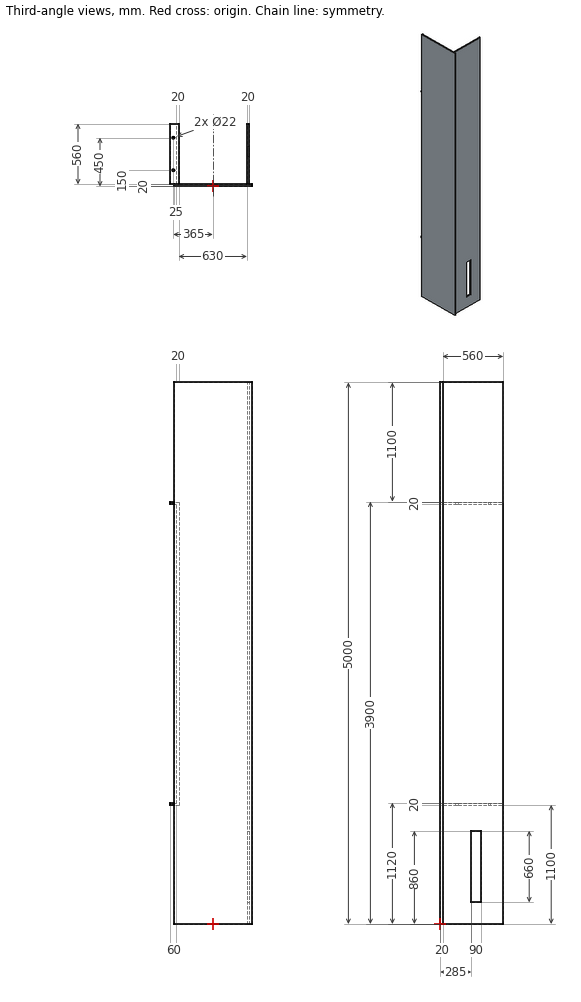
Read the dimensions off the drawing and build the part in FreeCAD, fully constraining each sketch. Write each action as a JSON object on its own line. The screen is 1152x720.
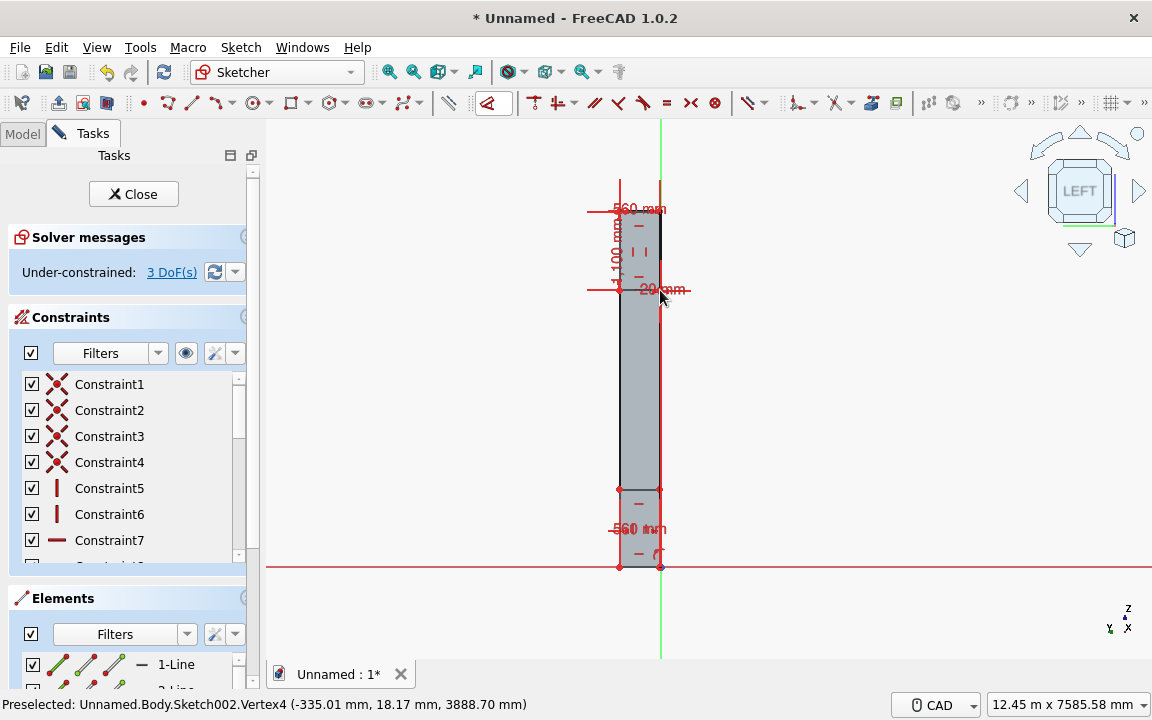
{"action": "scroll", "coordinate": [660, 567], "scroll_direction": "up", "scroll_amount": 17}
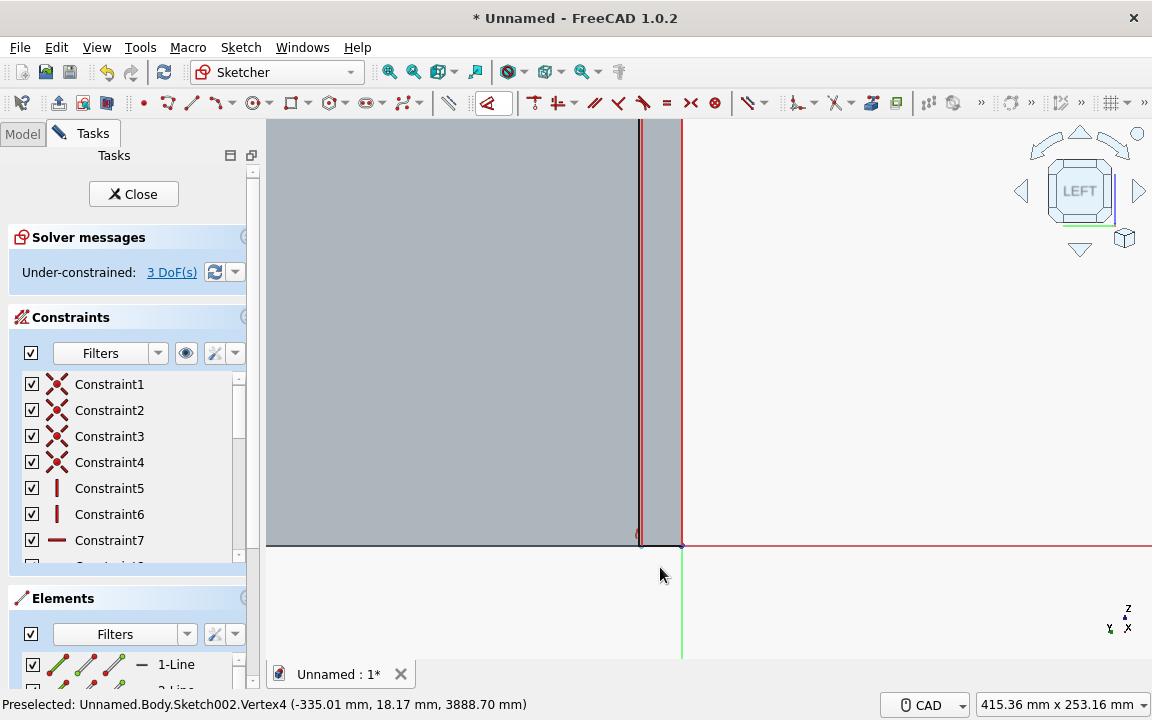
{"action": "left_click", "coordinate": [642, 546]}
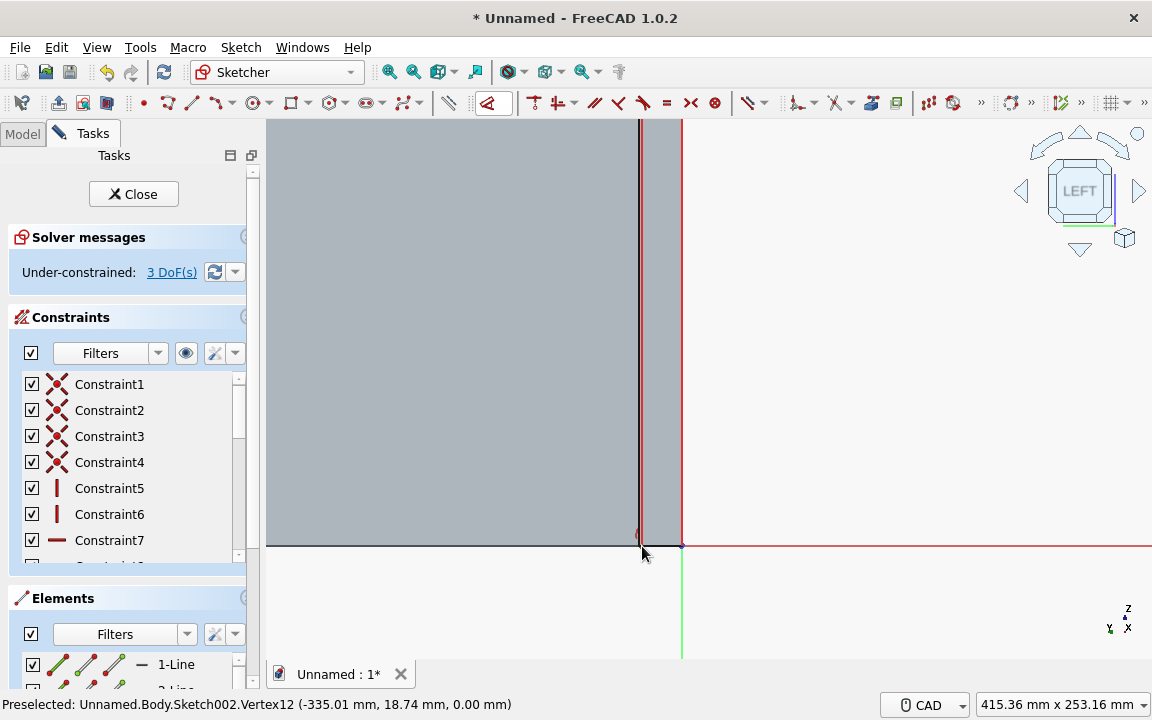
{"action": "left_click", "coordinate": [506, 104]}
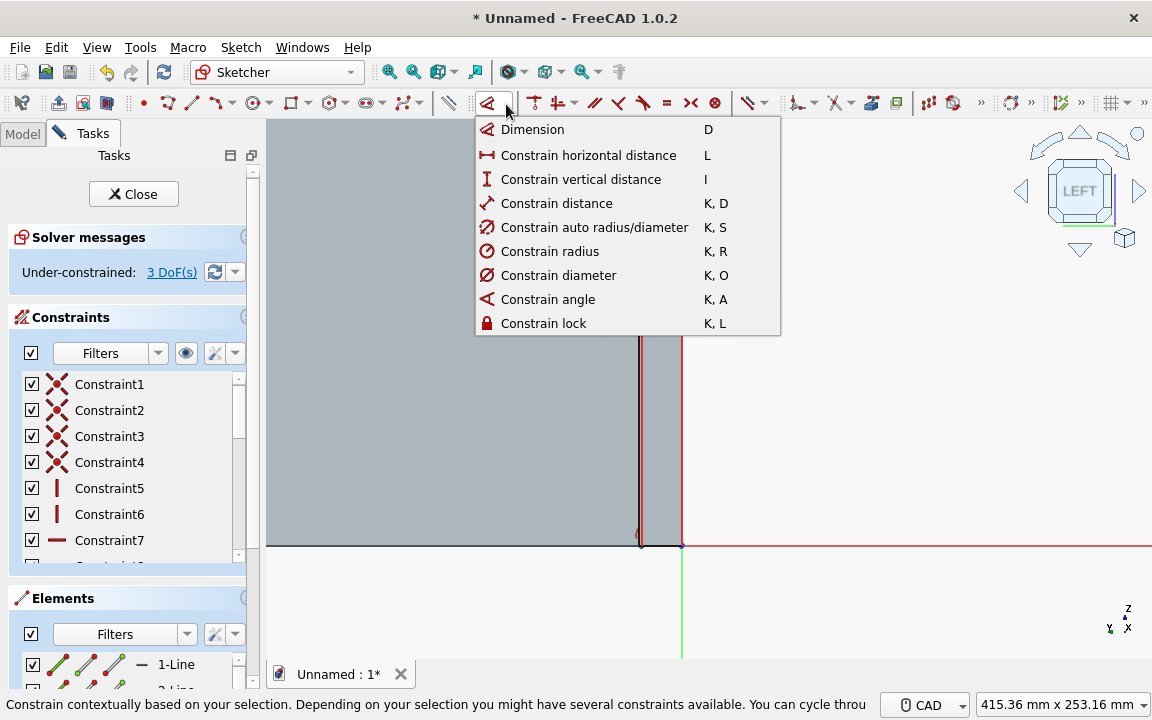
{"action": "left_click", "coordinate": [628, 155]}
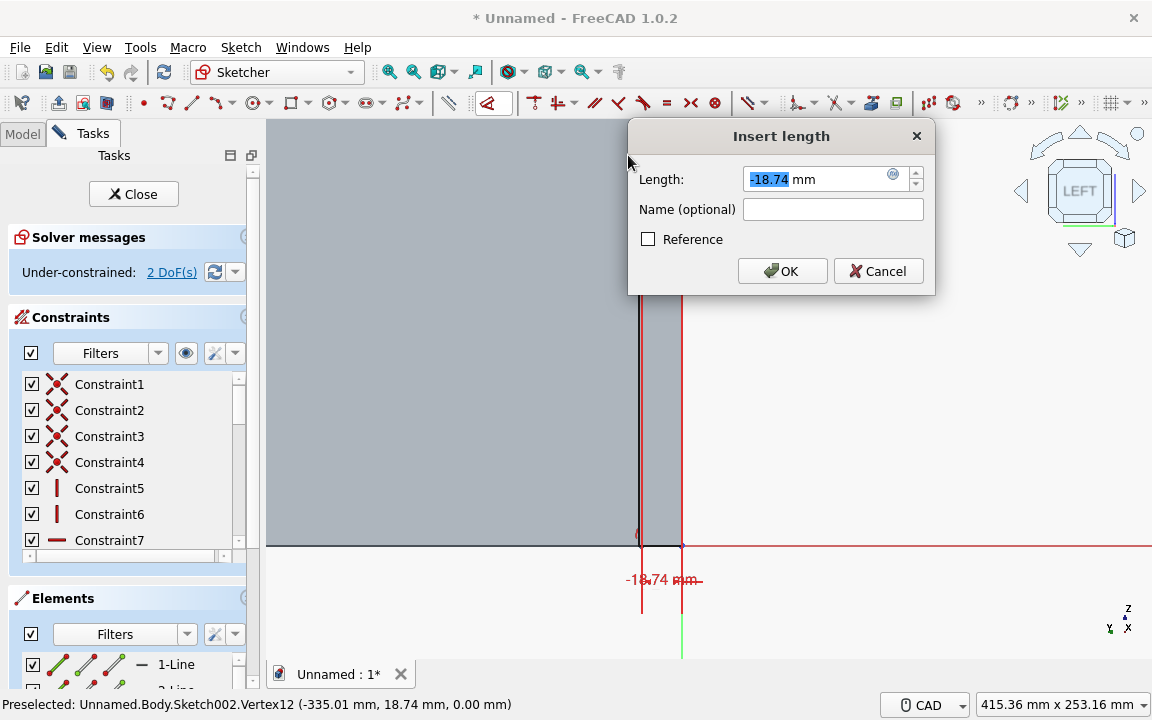
{"action": "type", "text": "-20"}
{"action": "key", "text": "Return"}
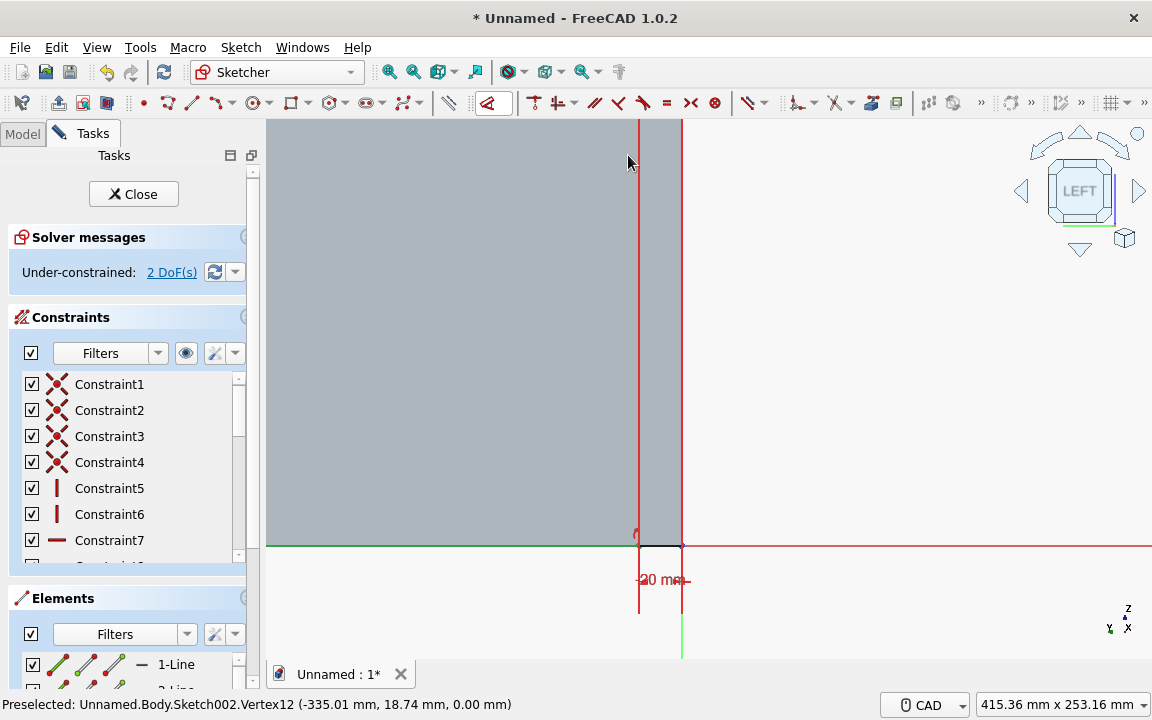
{"action": "scroll", "coordinate": [660, 568], "scroll_direction": "down", "scroll_amount": 17}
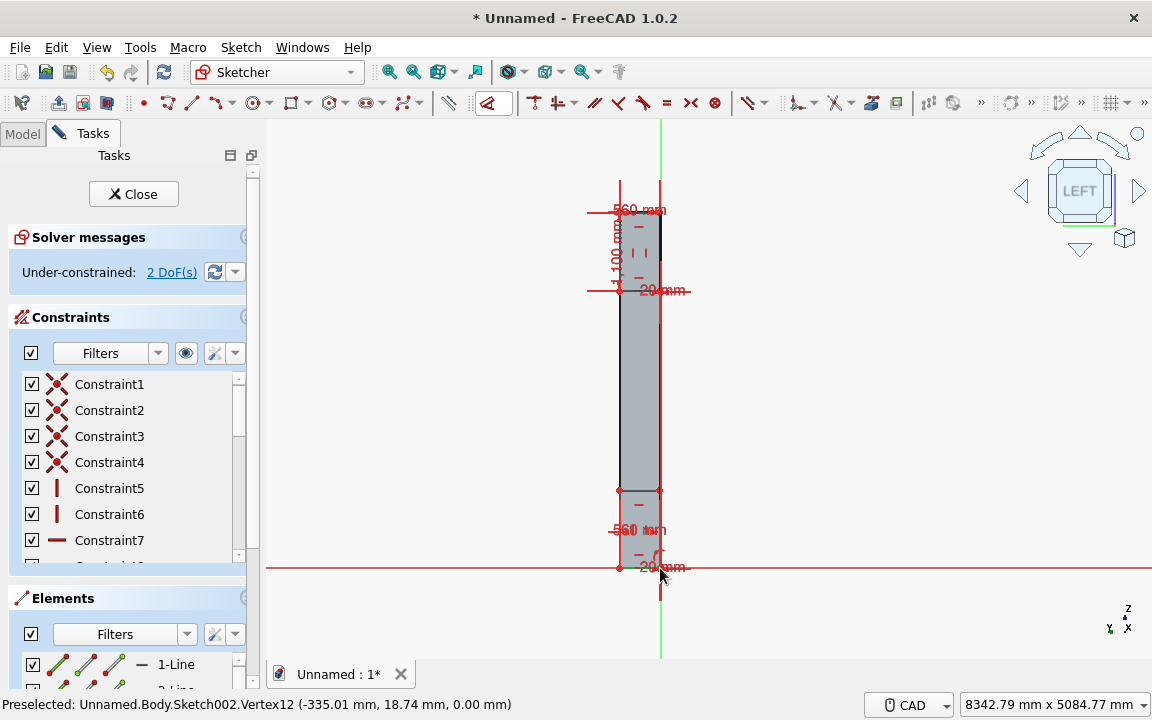
{"action": "left_click", "coordinate": [620, 514]}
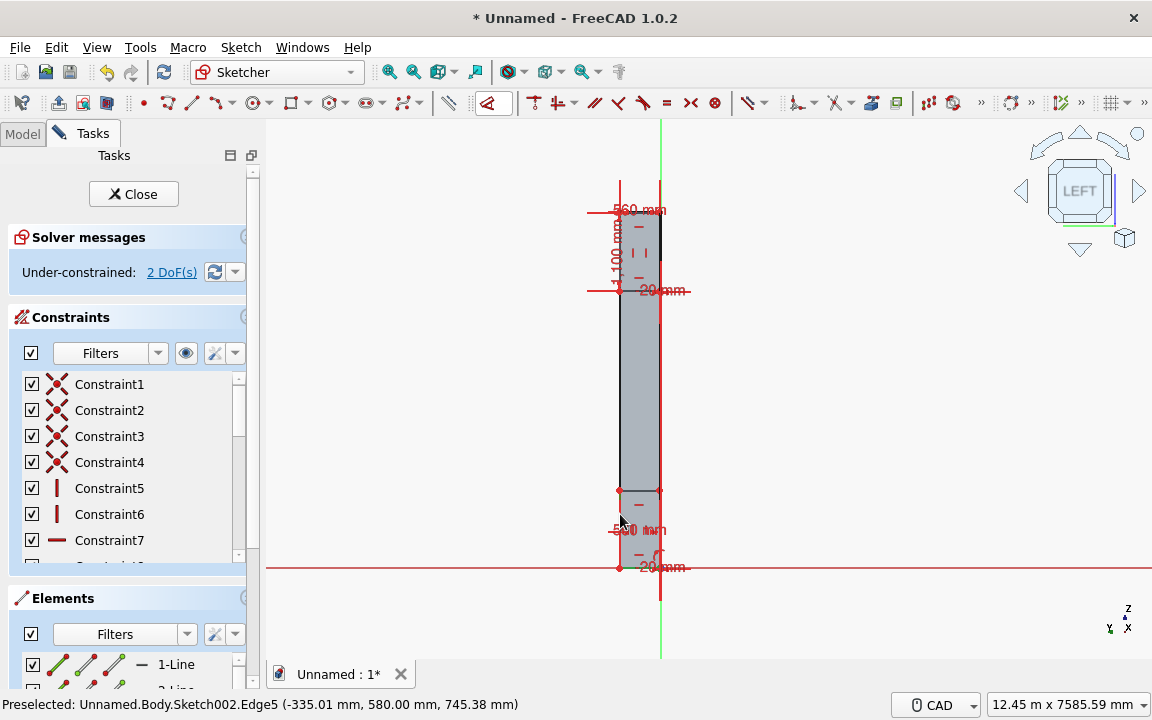
{"action": "key", "text": "i"}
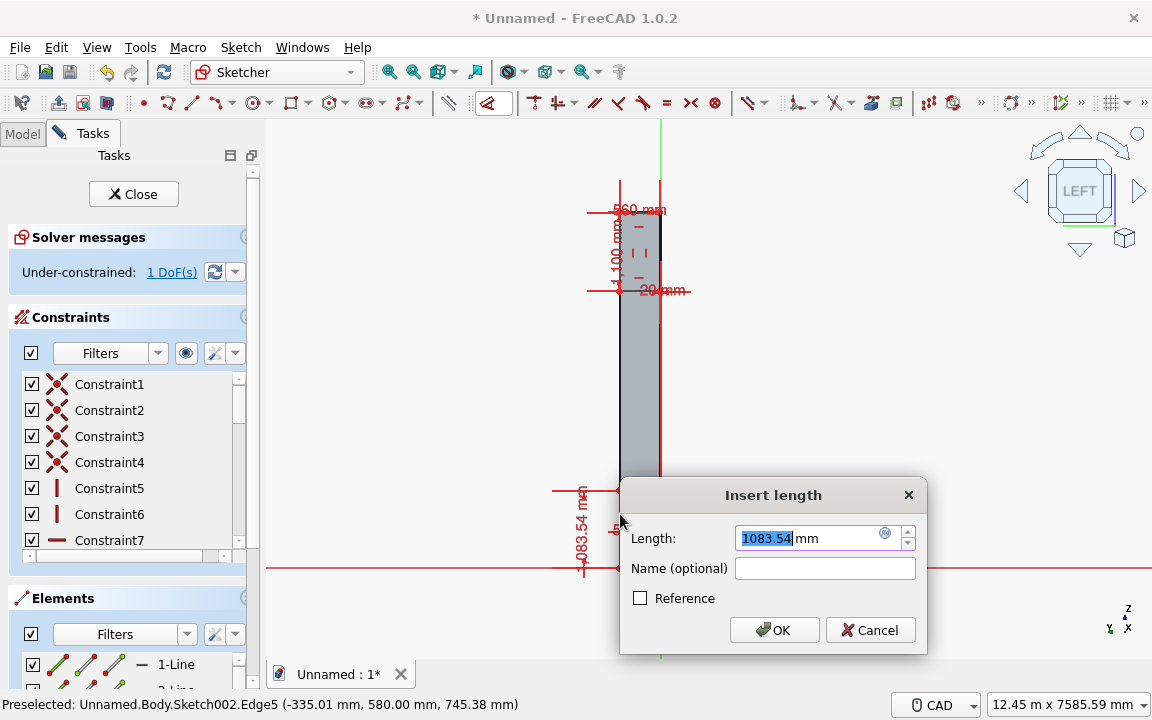
{"action": "type", "text": "1100"}
{"action": "key", "text": "Return"}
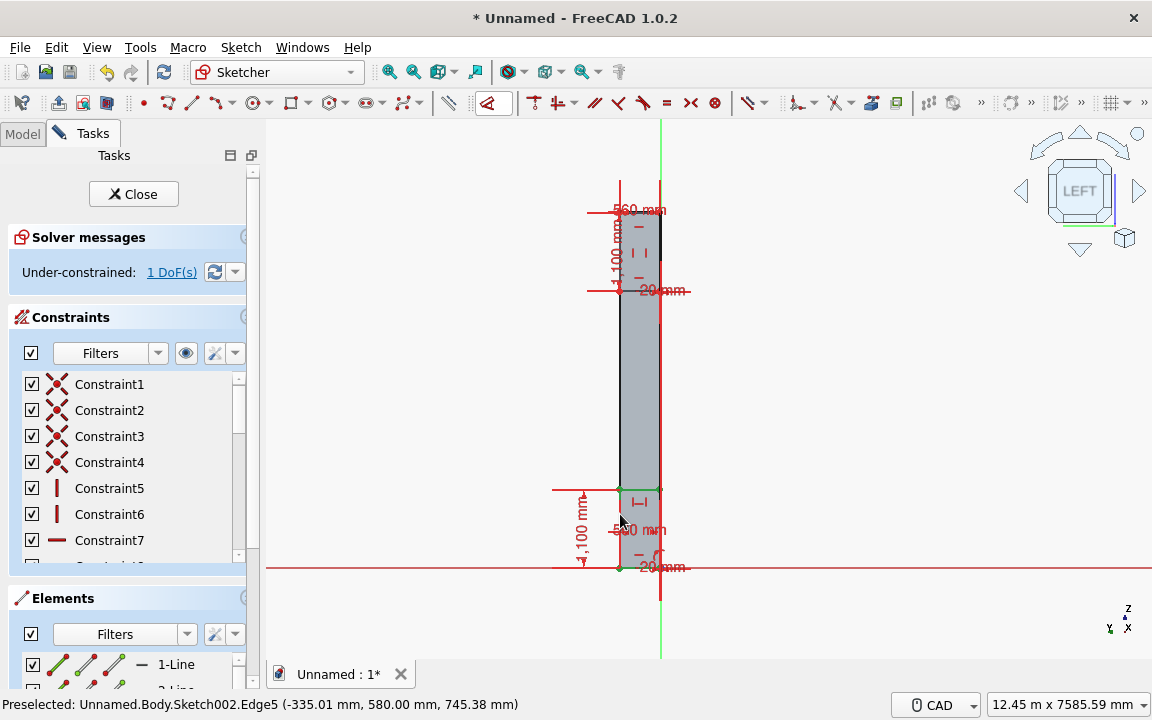
{"action": "left_click", "coordinate": [620, 213]}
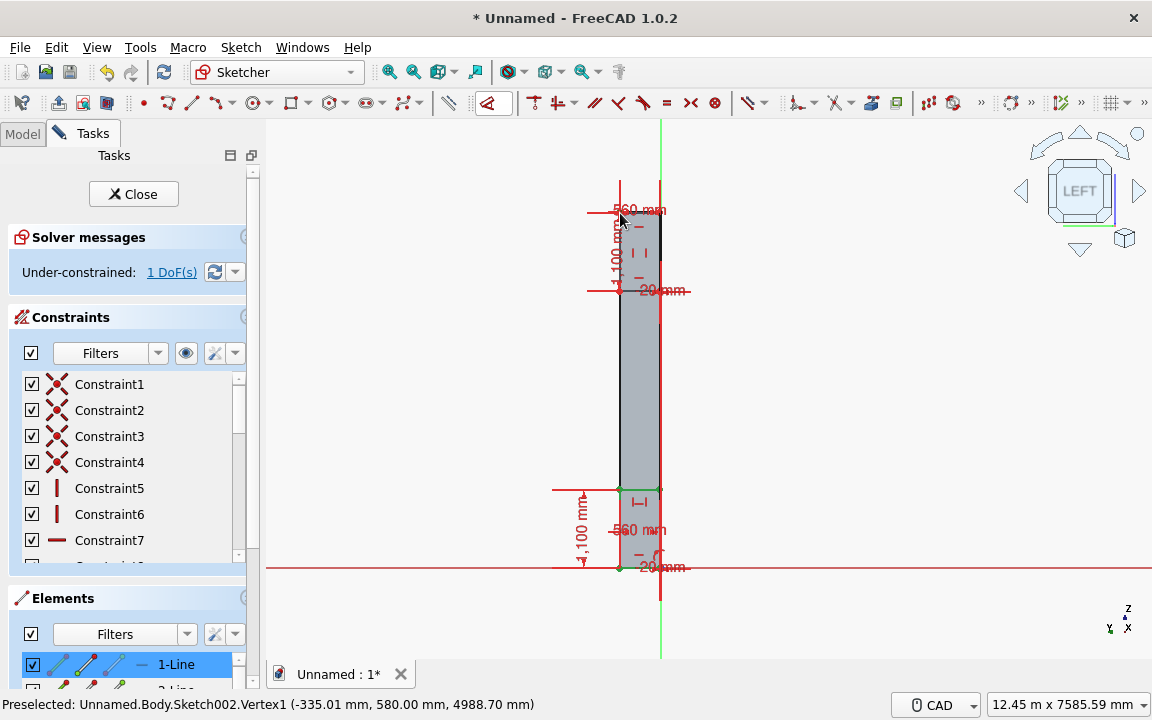
{"action": "key", "text": "i"}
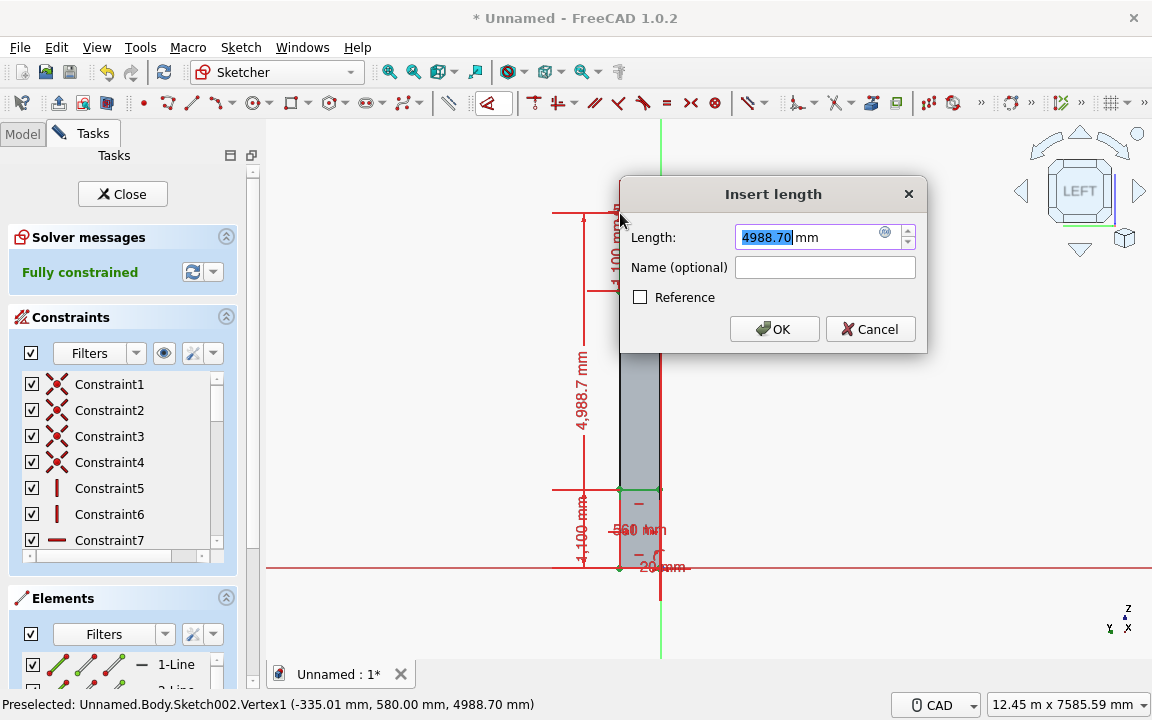
{"action": "type", "text": "5000"}
{"action": "key", "text": "Return"}